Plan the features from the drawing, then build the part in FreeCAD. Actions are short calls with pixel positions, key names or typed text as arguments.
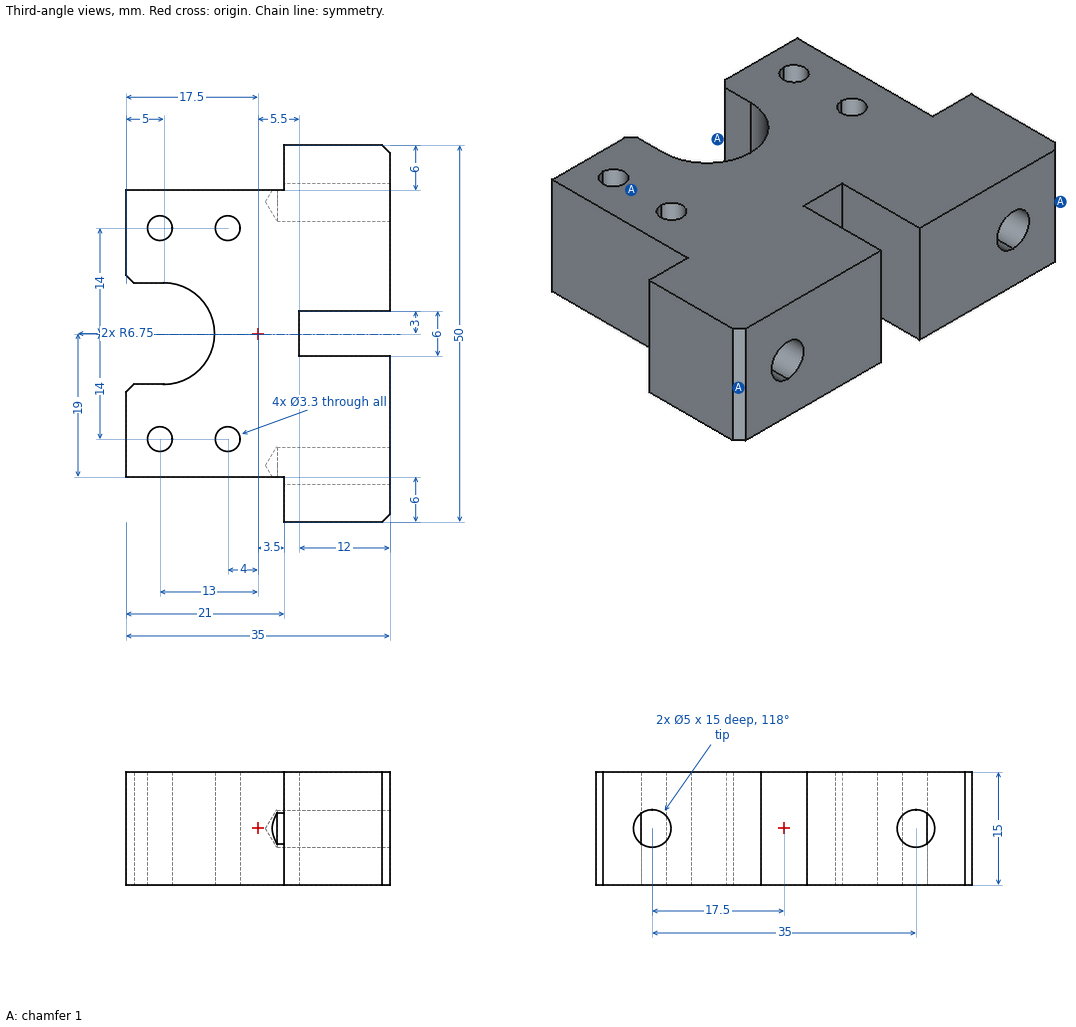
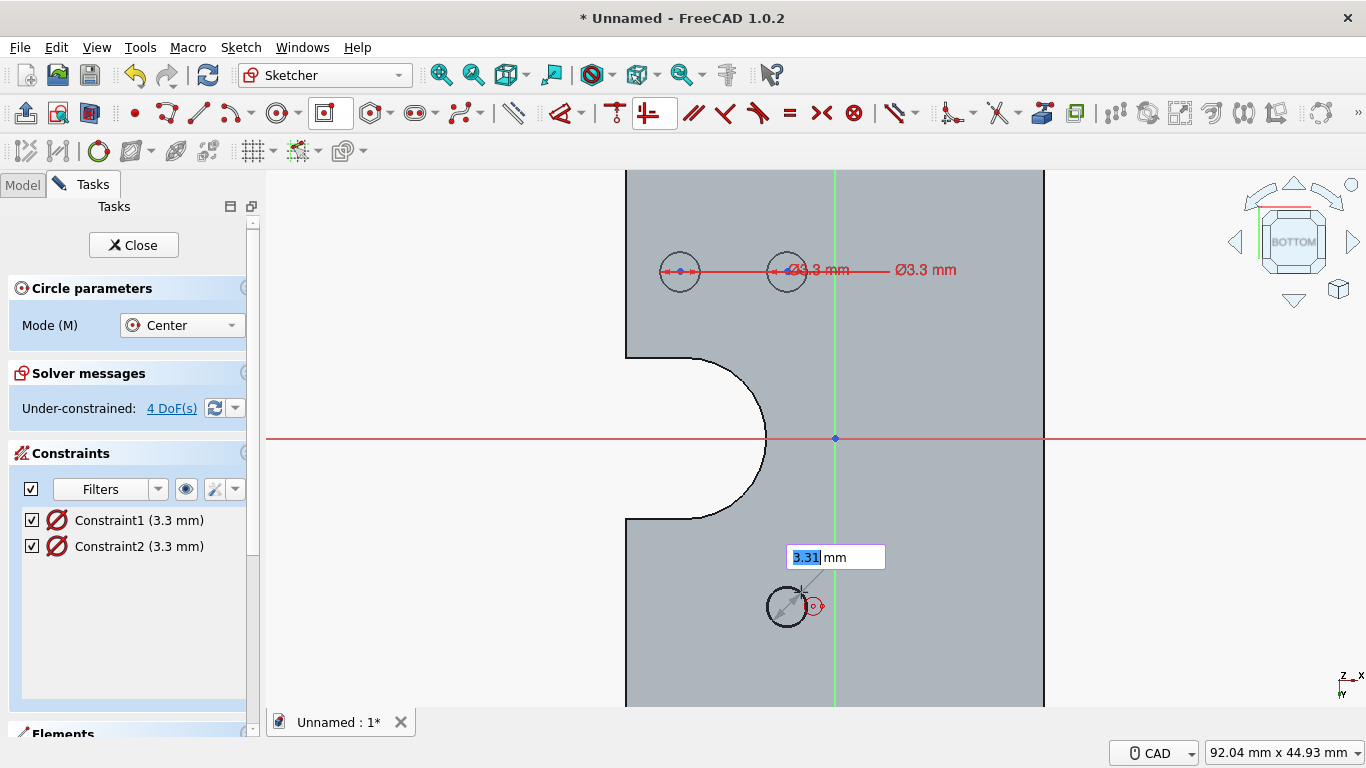
text(3.3)
key(Return)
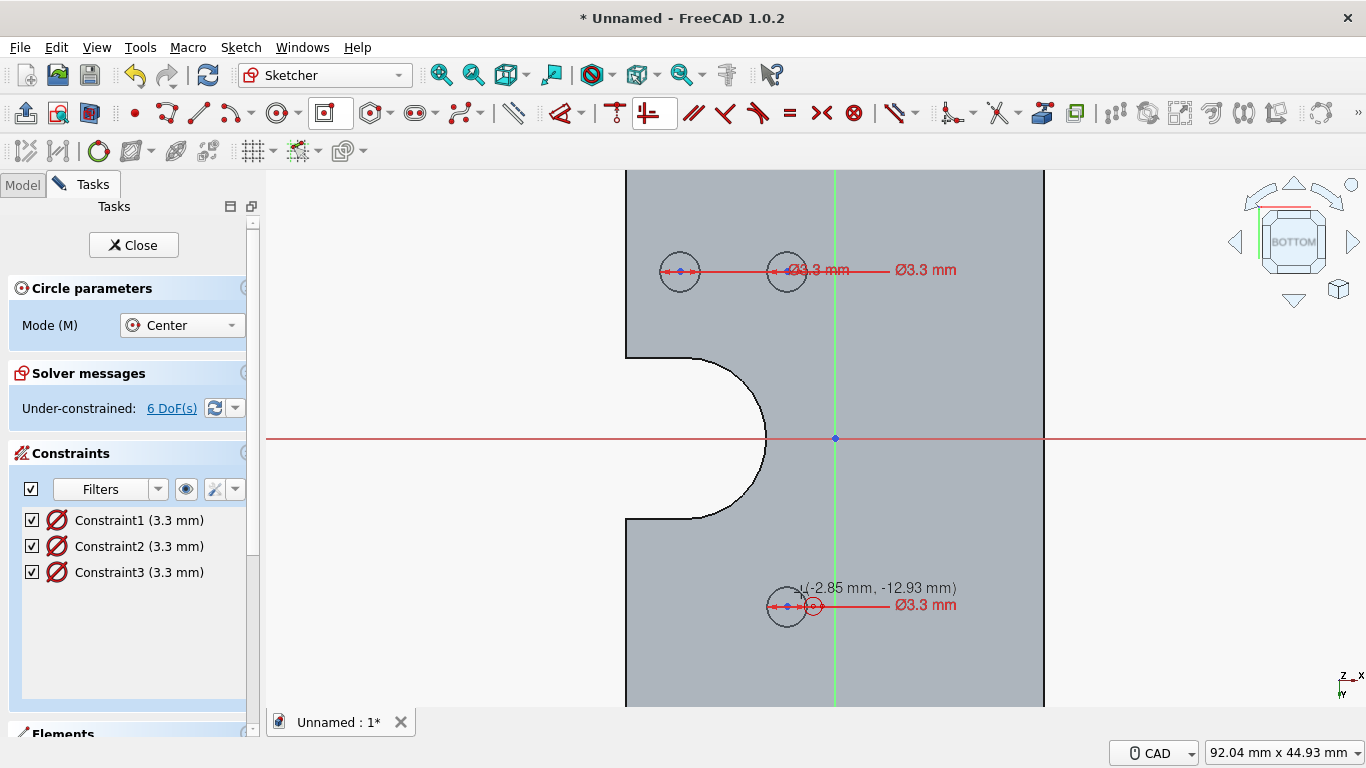
click(680, 606)
move(694, 592)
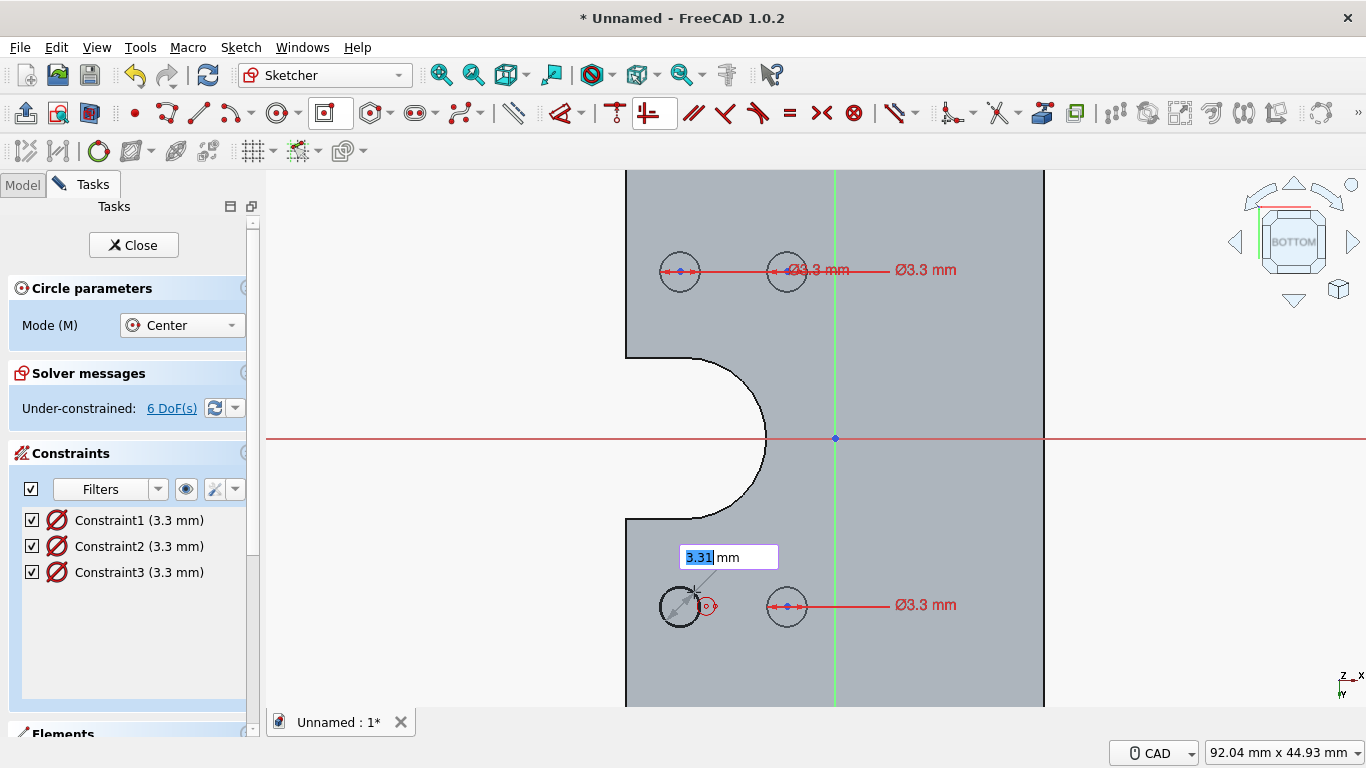
text(3.3)
key(Return)
key(Escape)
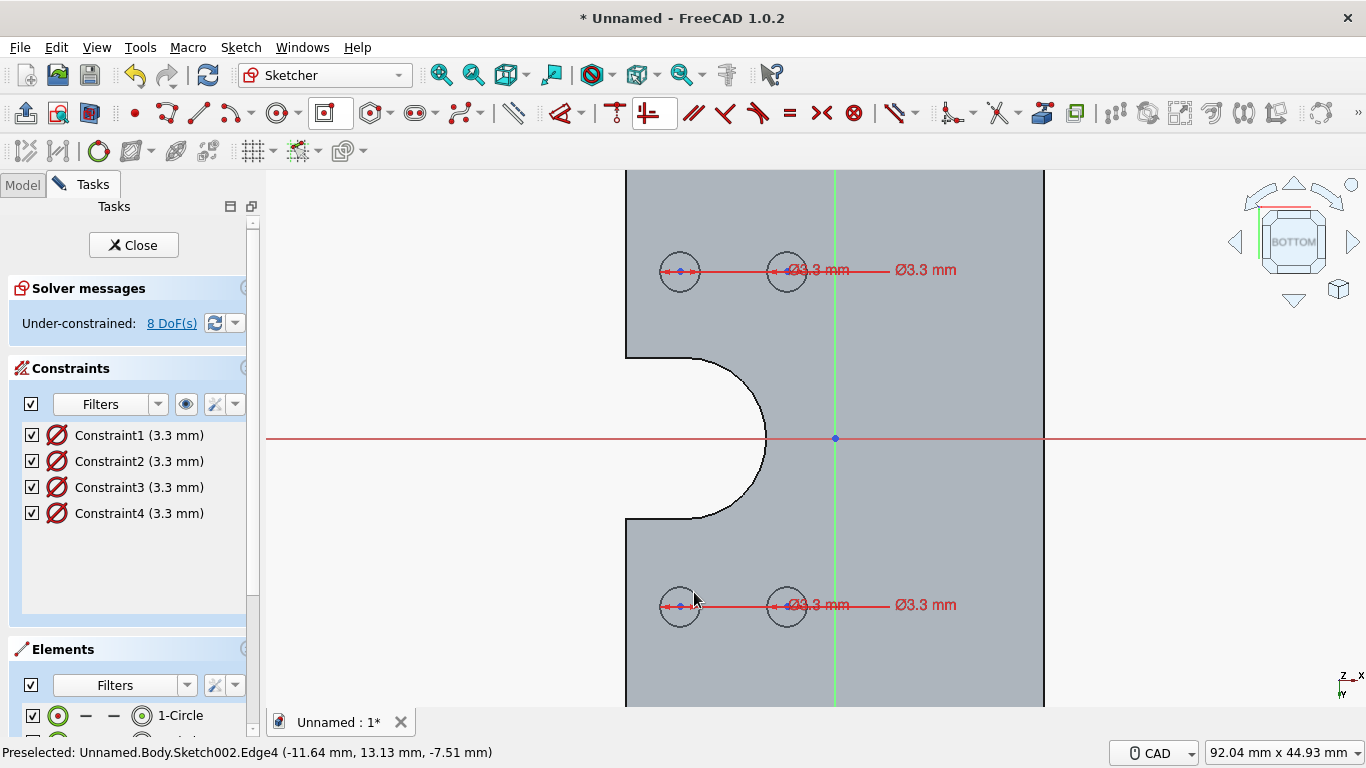
click(787, 272)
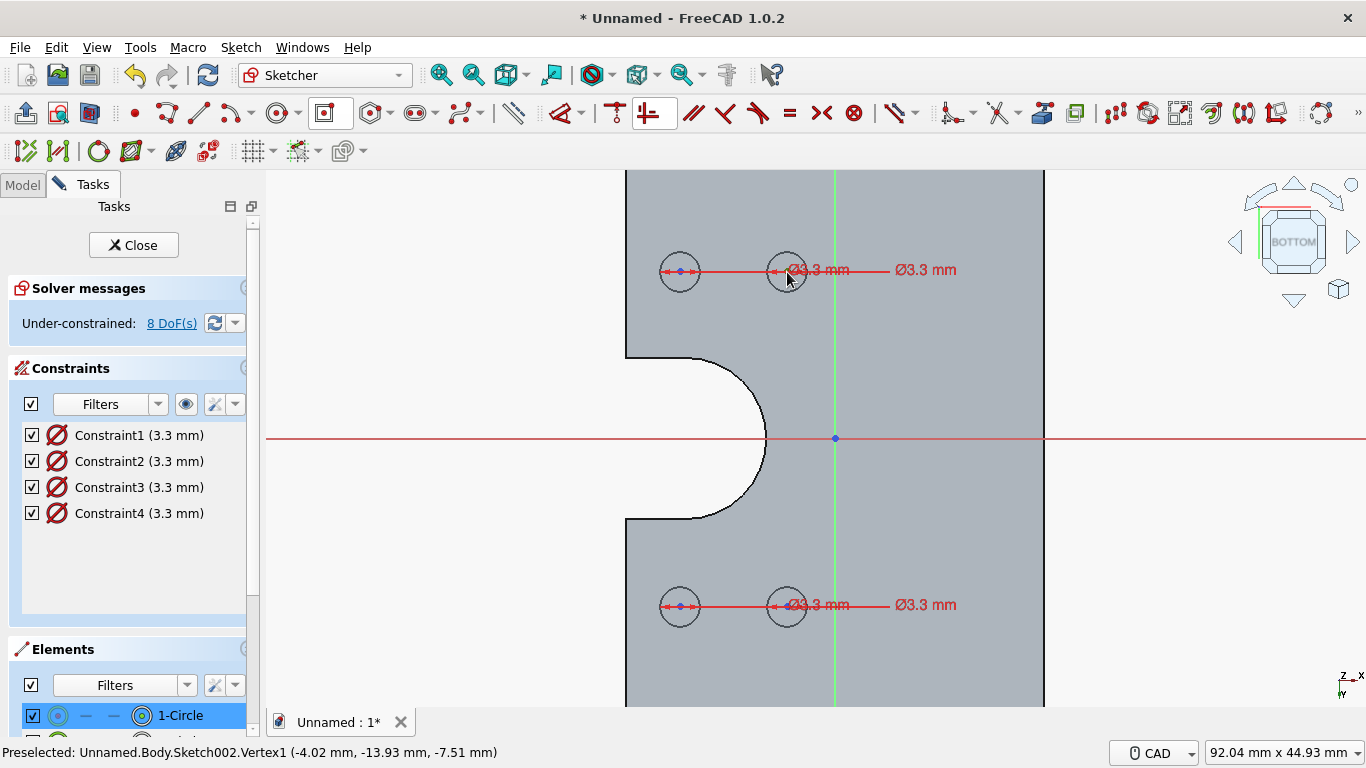
click(680, 272)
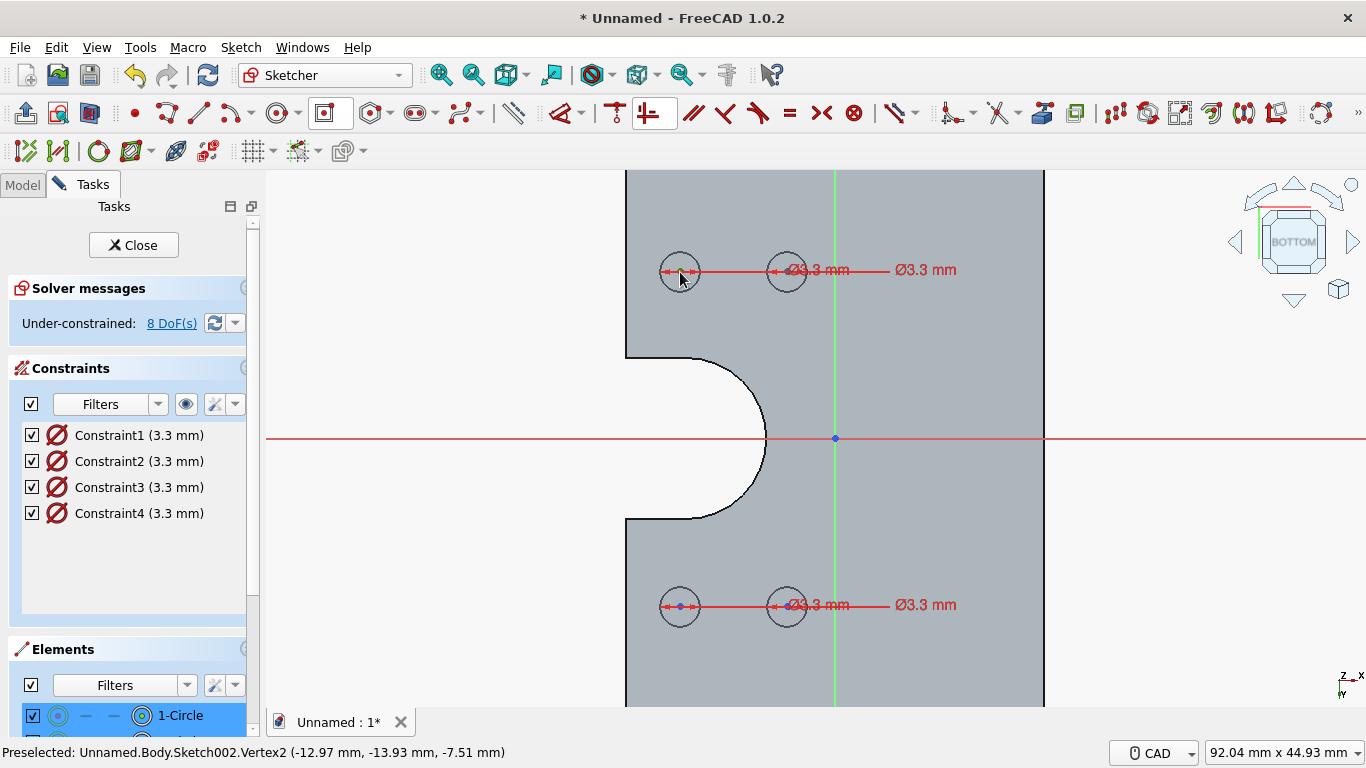
click(672, 114)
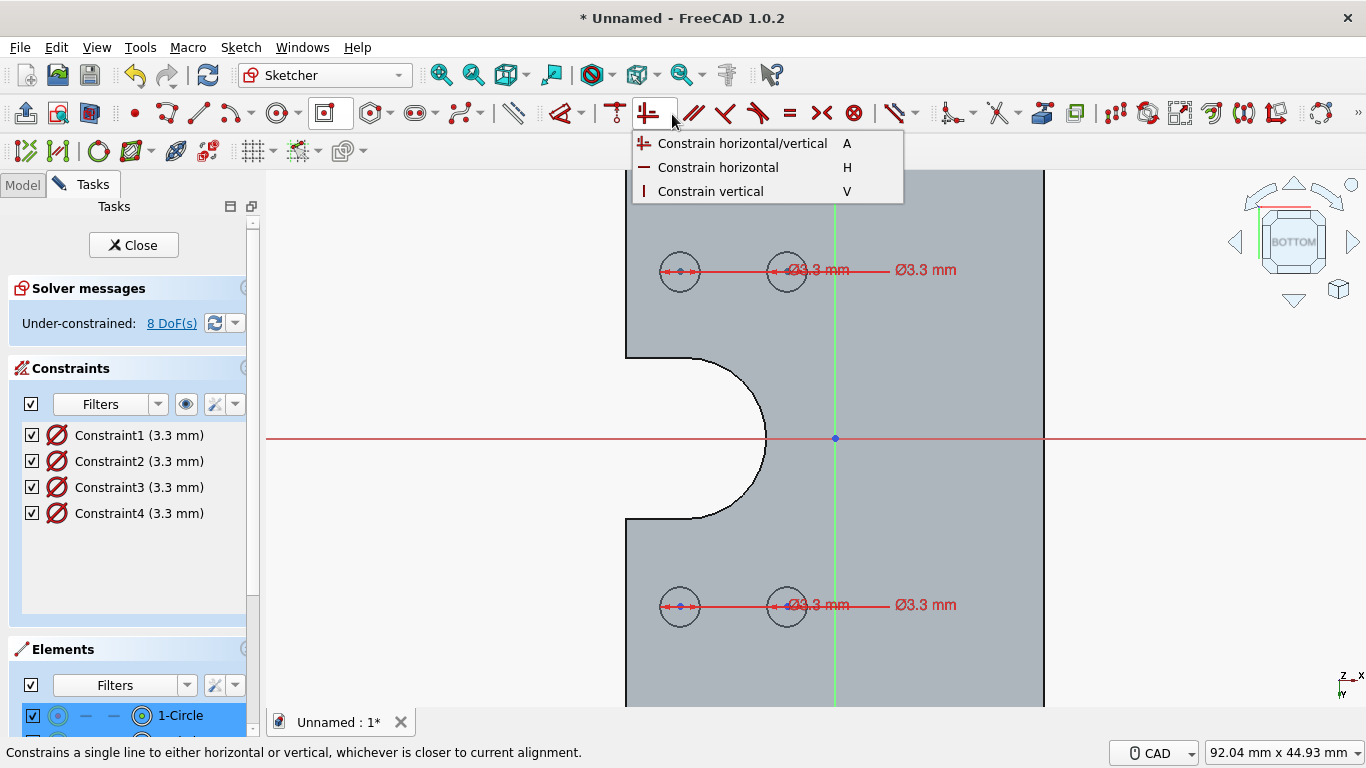
click(768, 167)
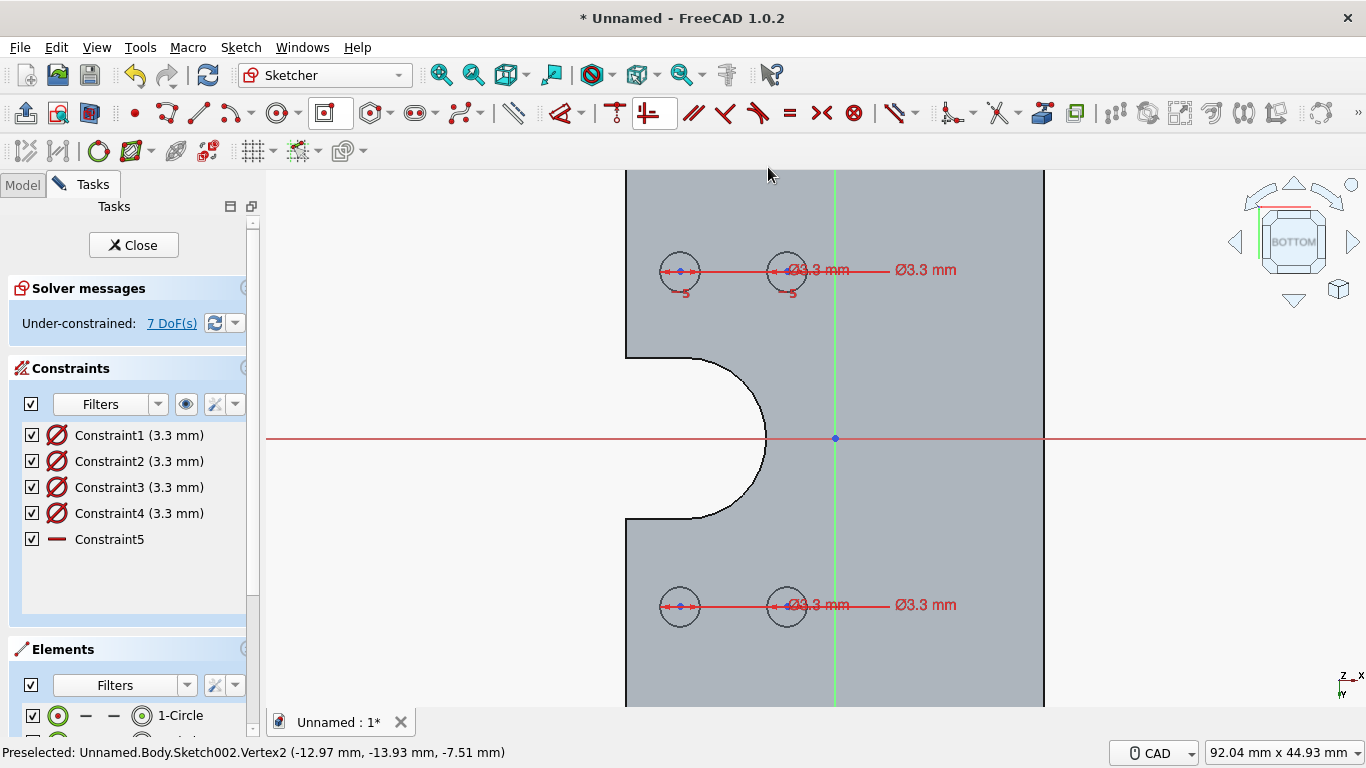
click(787, 272)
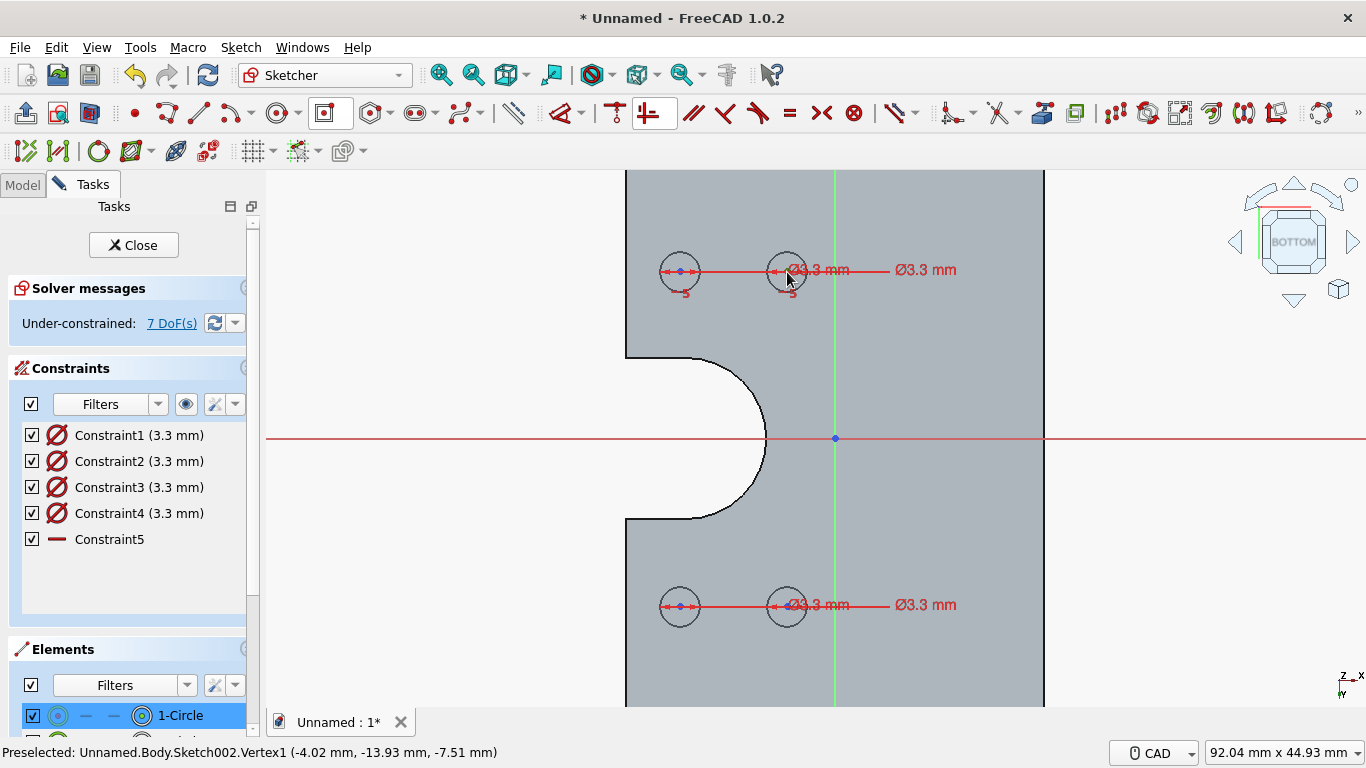
click(787, 607)